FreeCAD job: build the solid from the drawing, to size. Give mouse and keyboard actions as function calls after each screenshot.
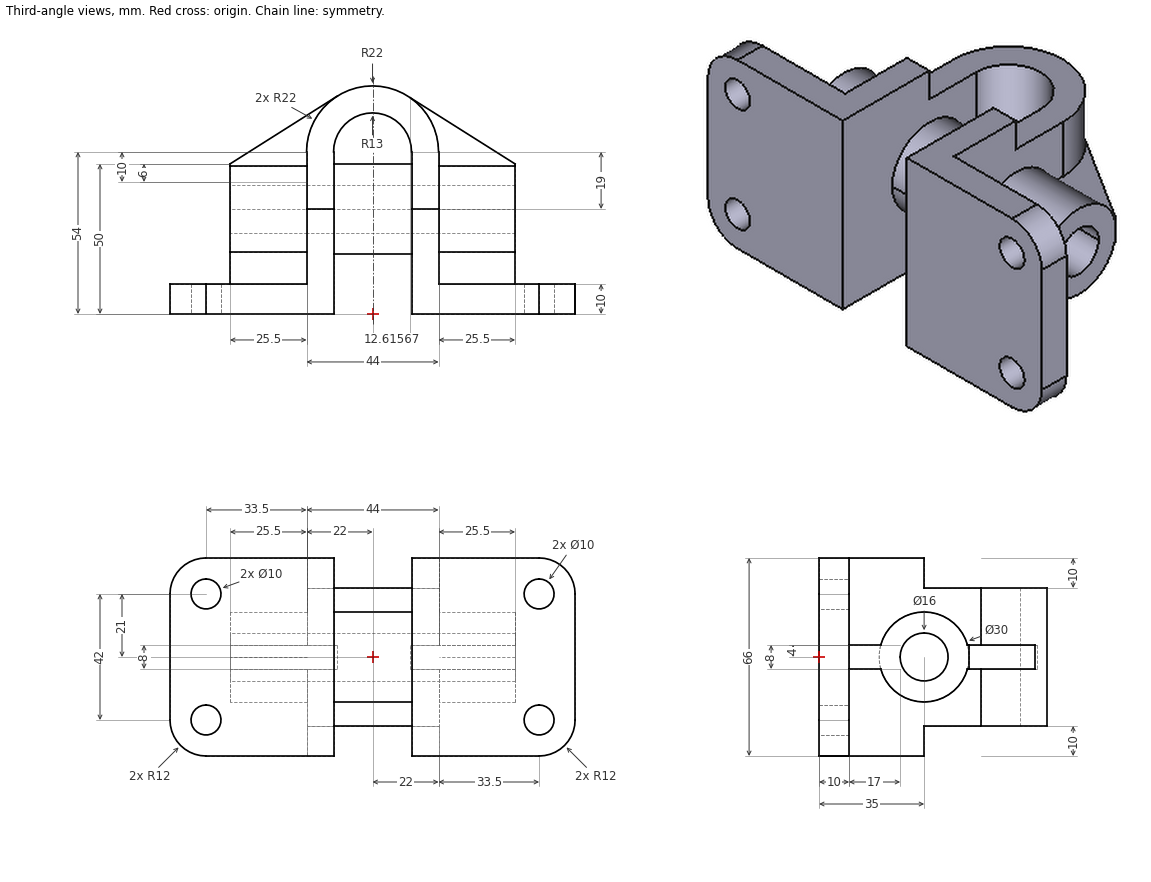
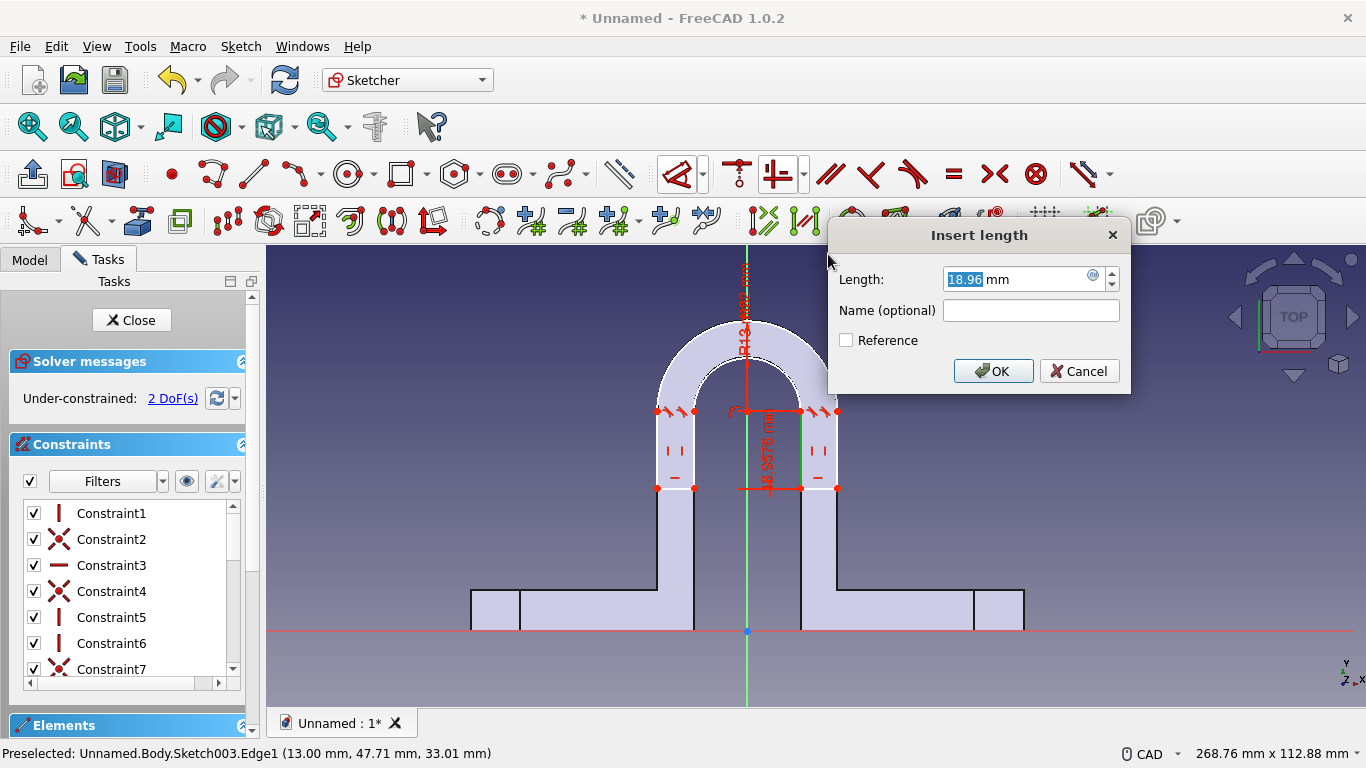
text(19)
key(Return)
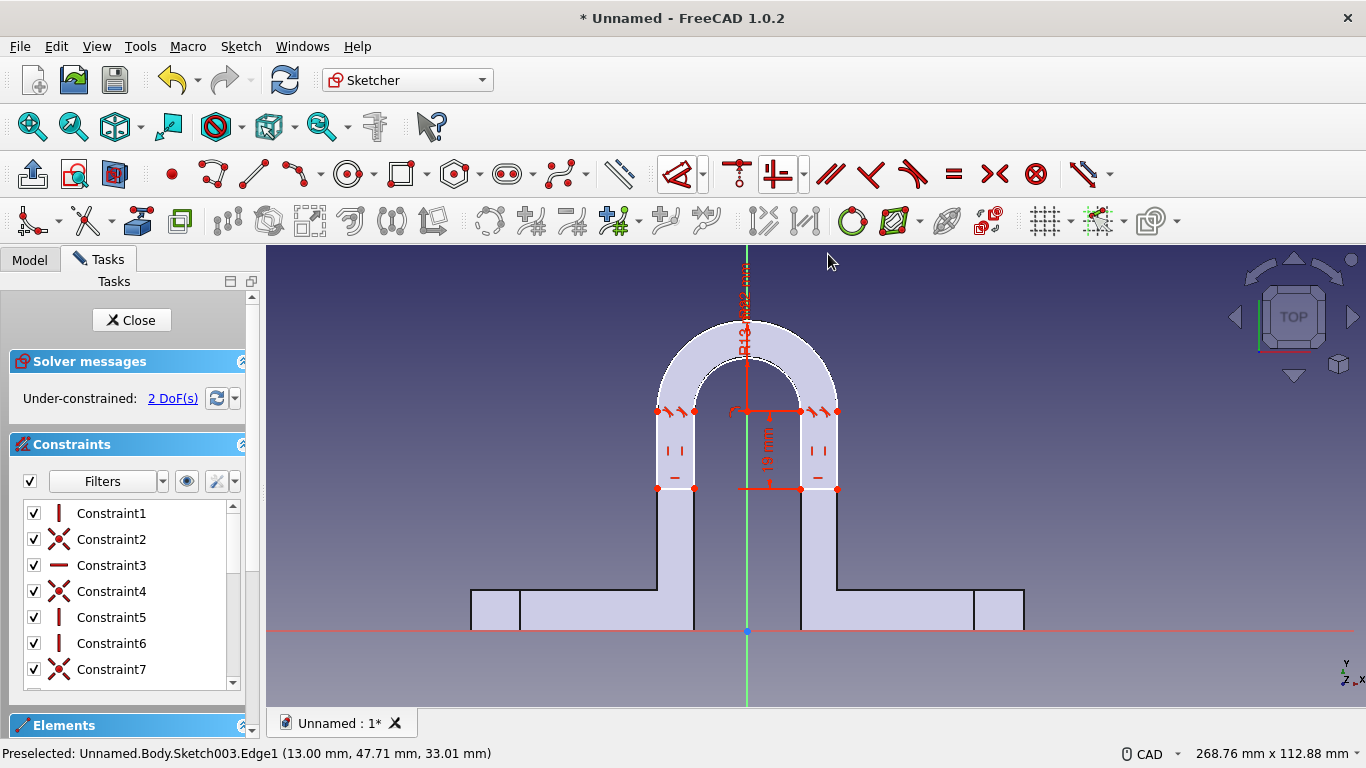
click(657, 435)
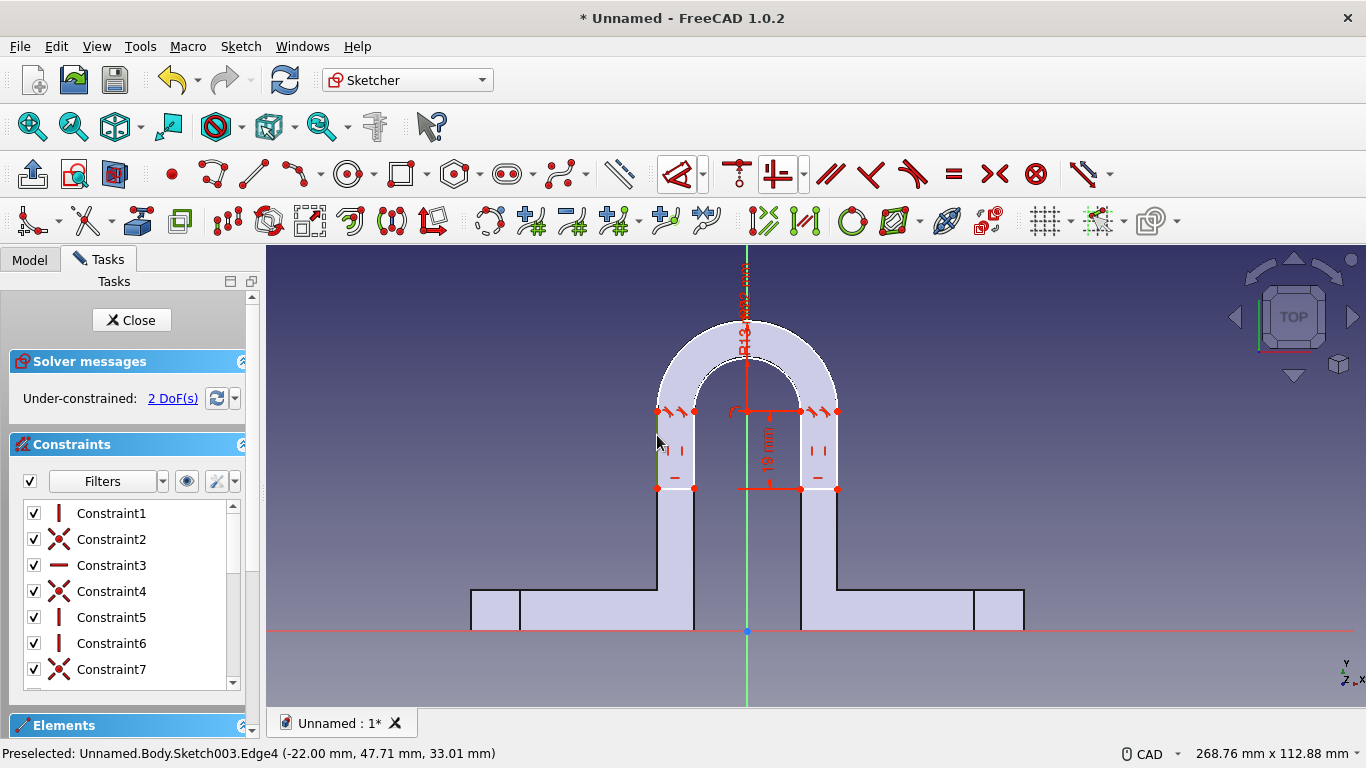
click(702, 174)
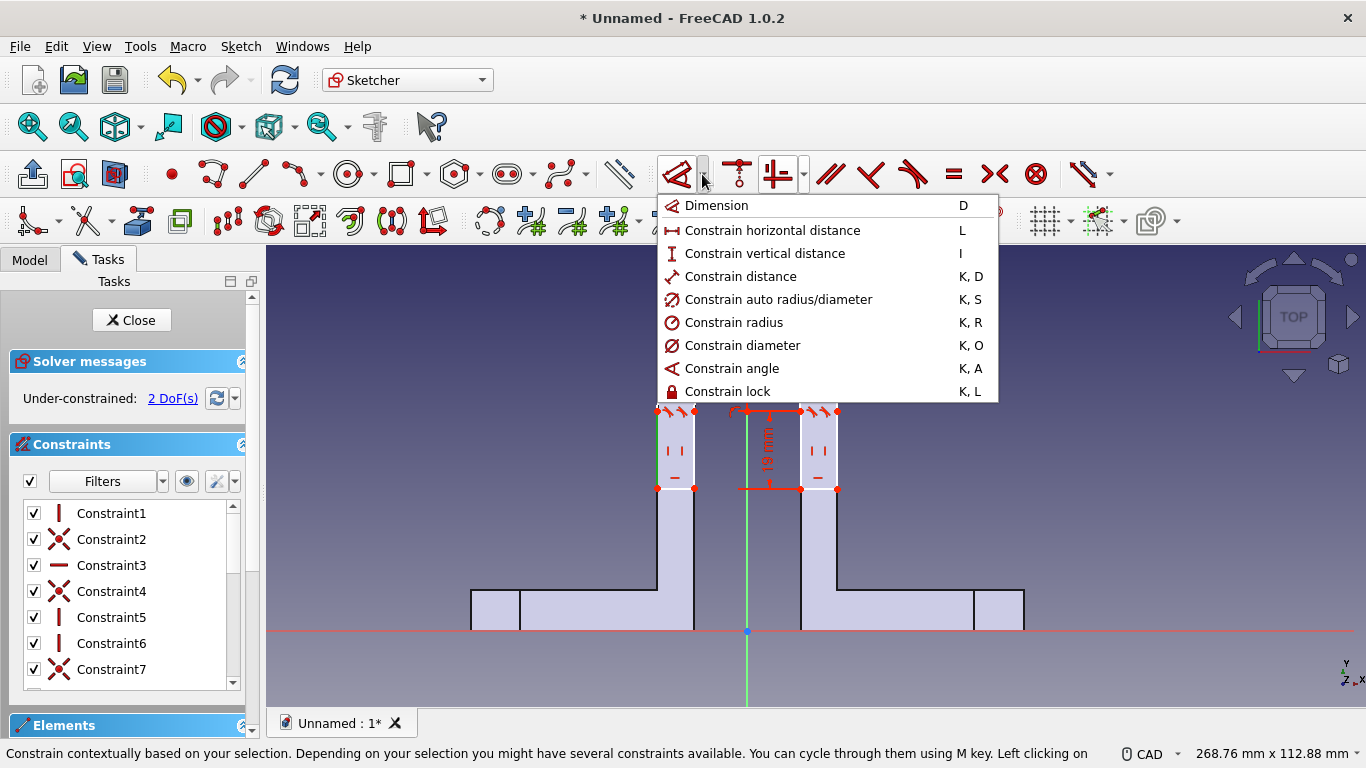
click(828, 254)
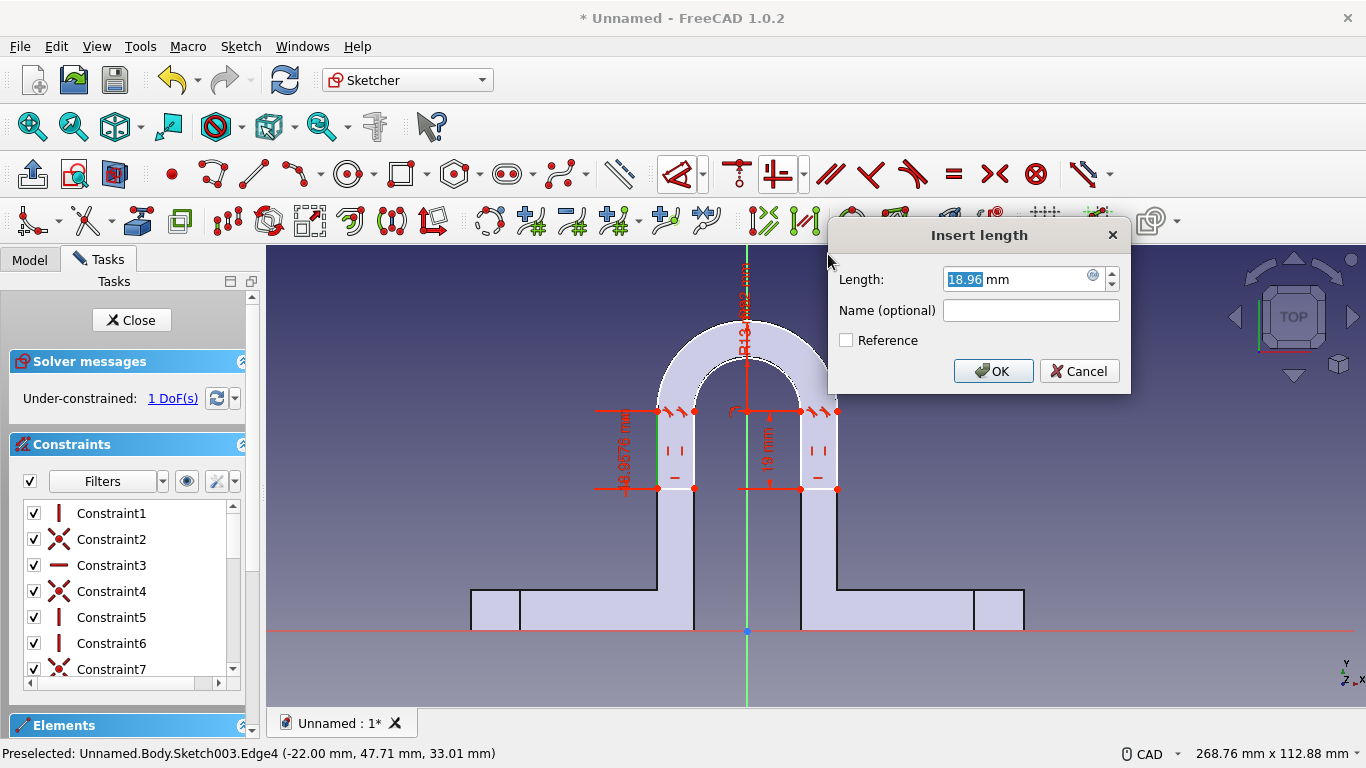
text(19)
key(Return)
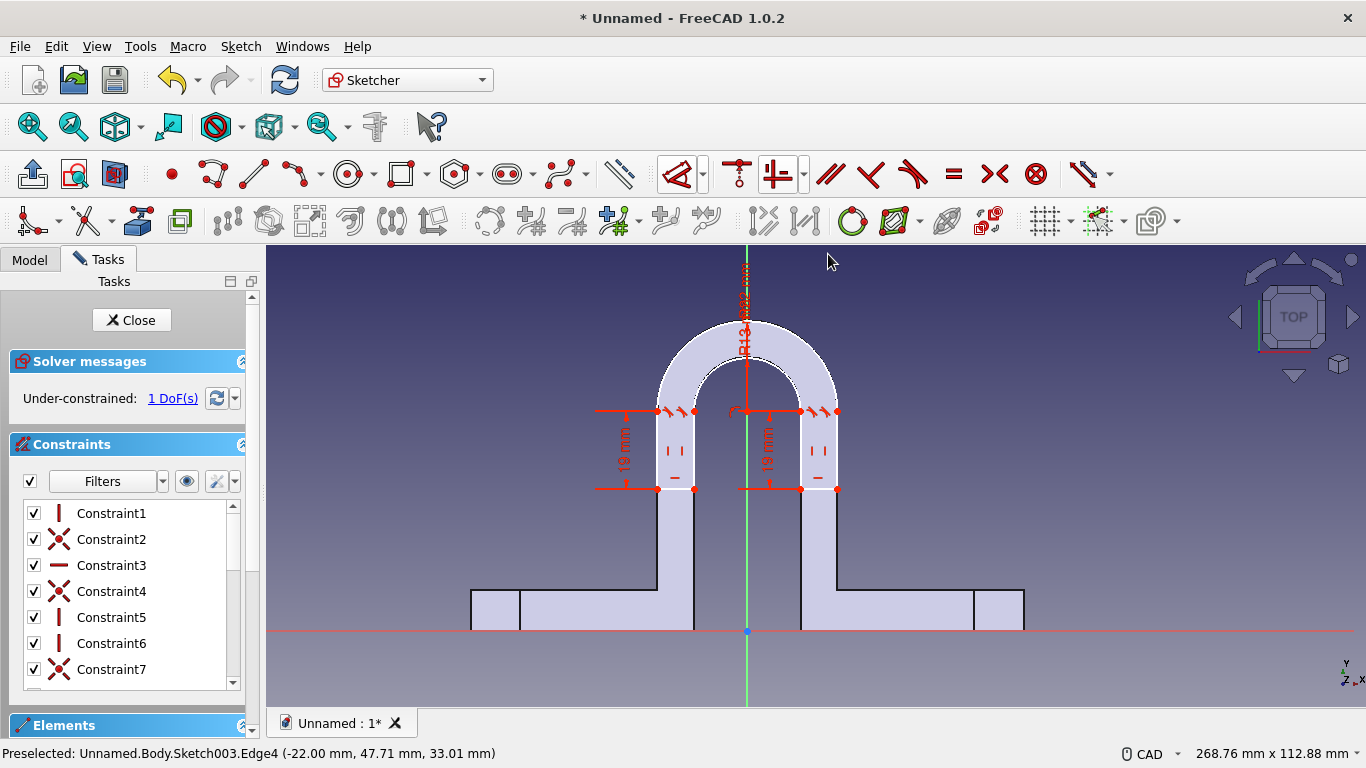
click(801, 411)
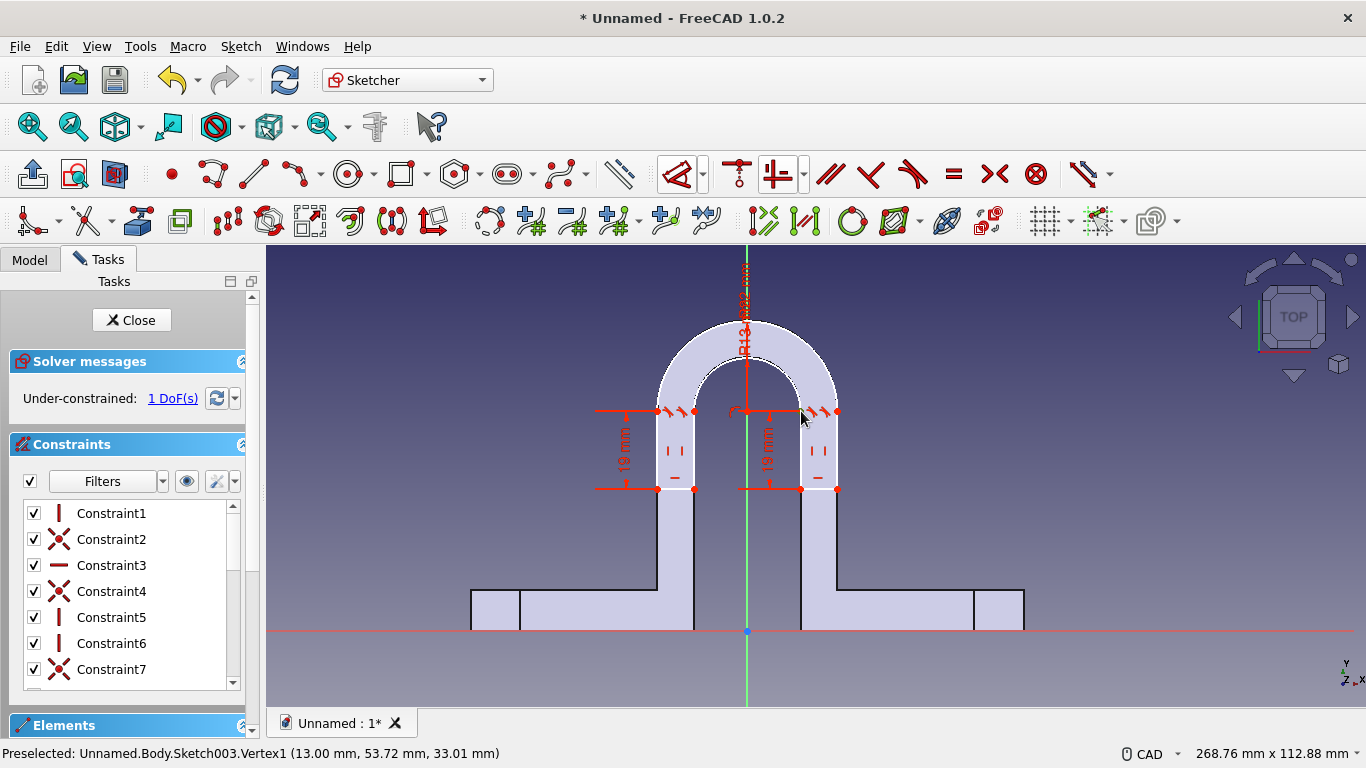
click(702, 174)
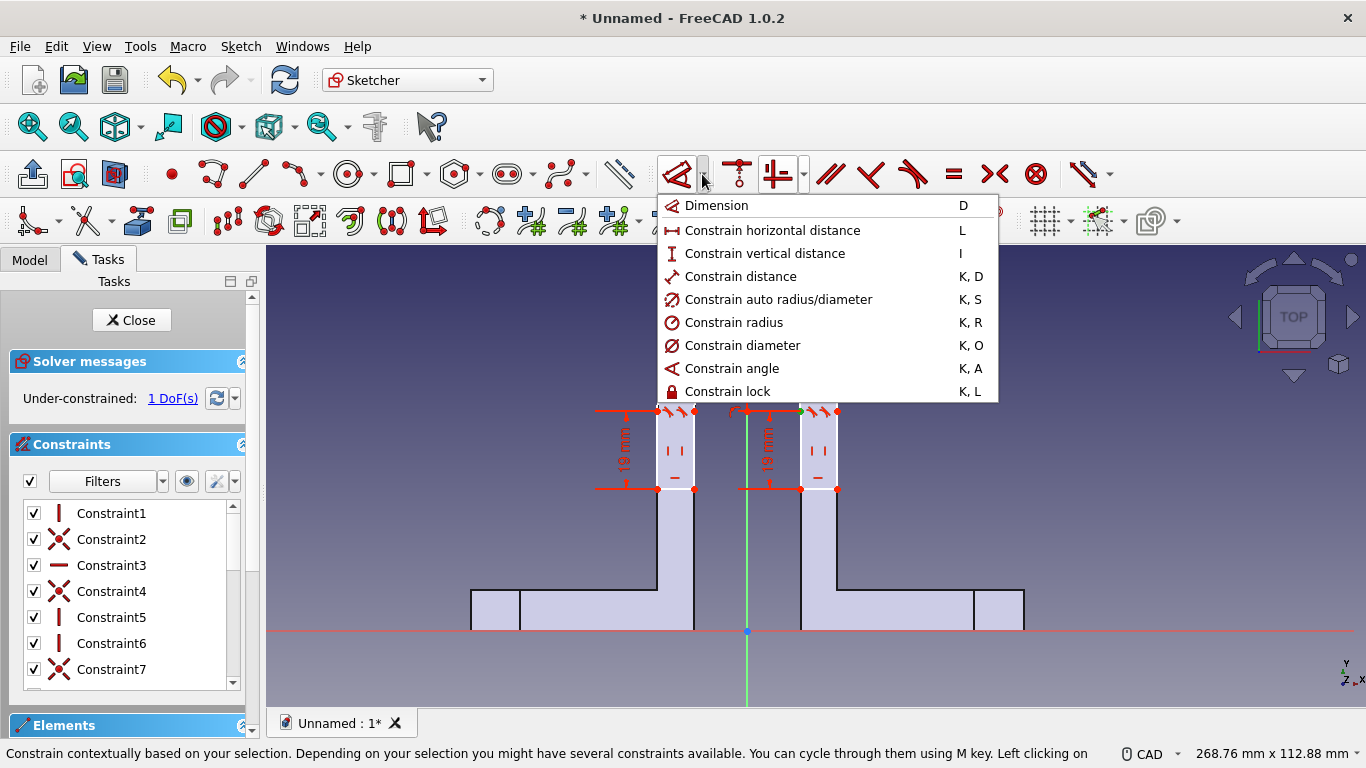
click(828, 254)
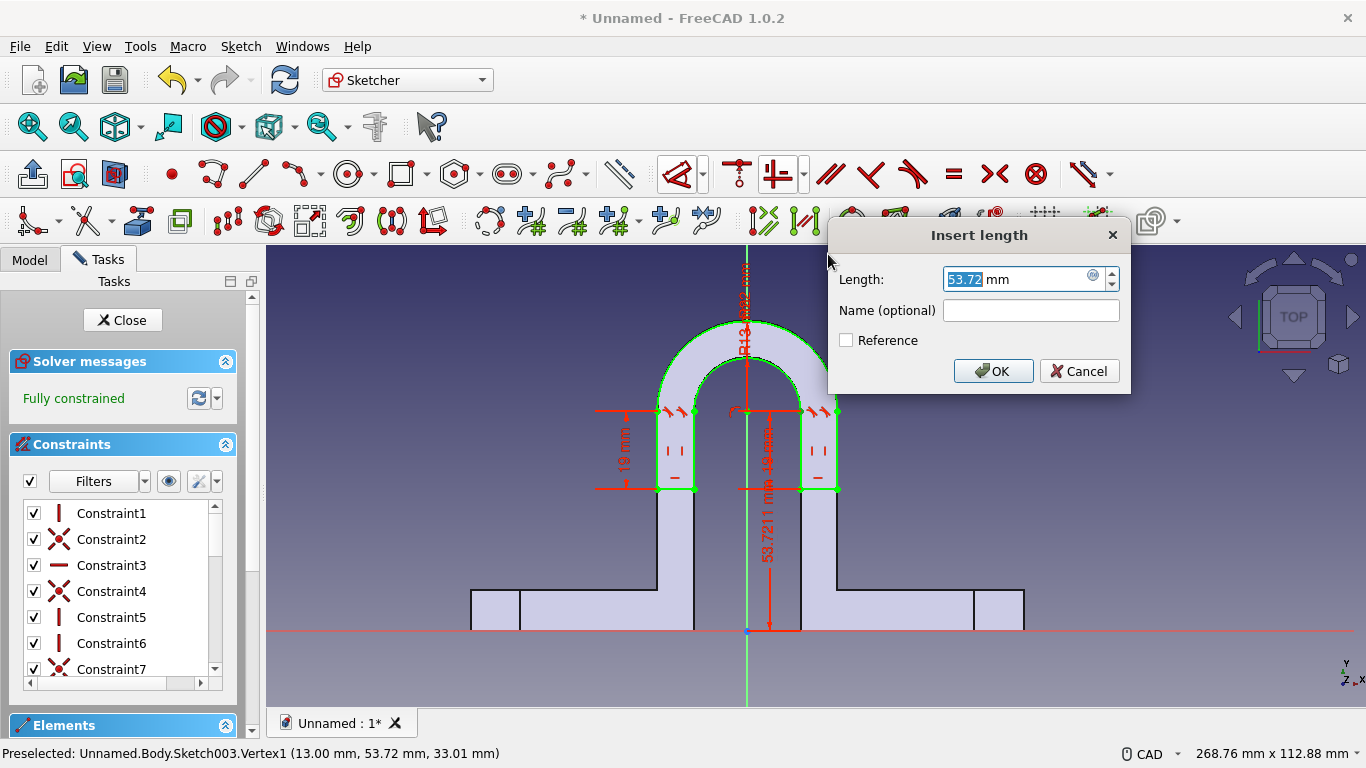
text(54)
key(Return)